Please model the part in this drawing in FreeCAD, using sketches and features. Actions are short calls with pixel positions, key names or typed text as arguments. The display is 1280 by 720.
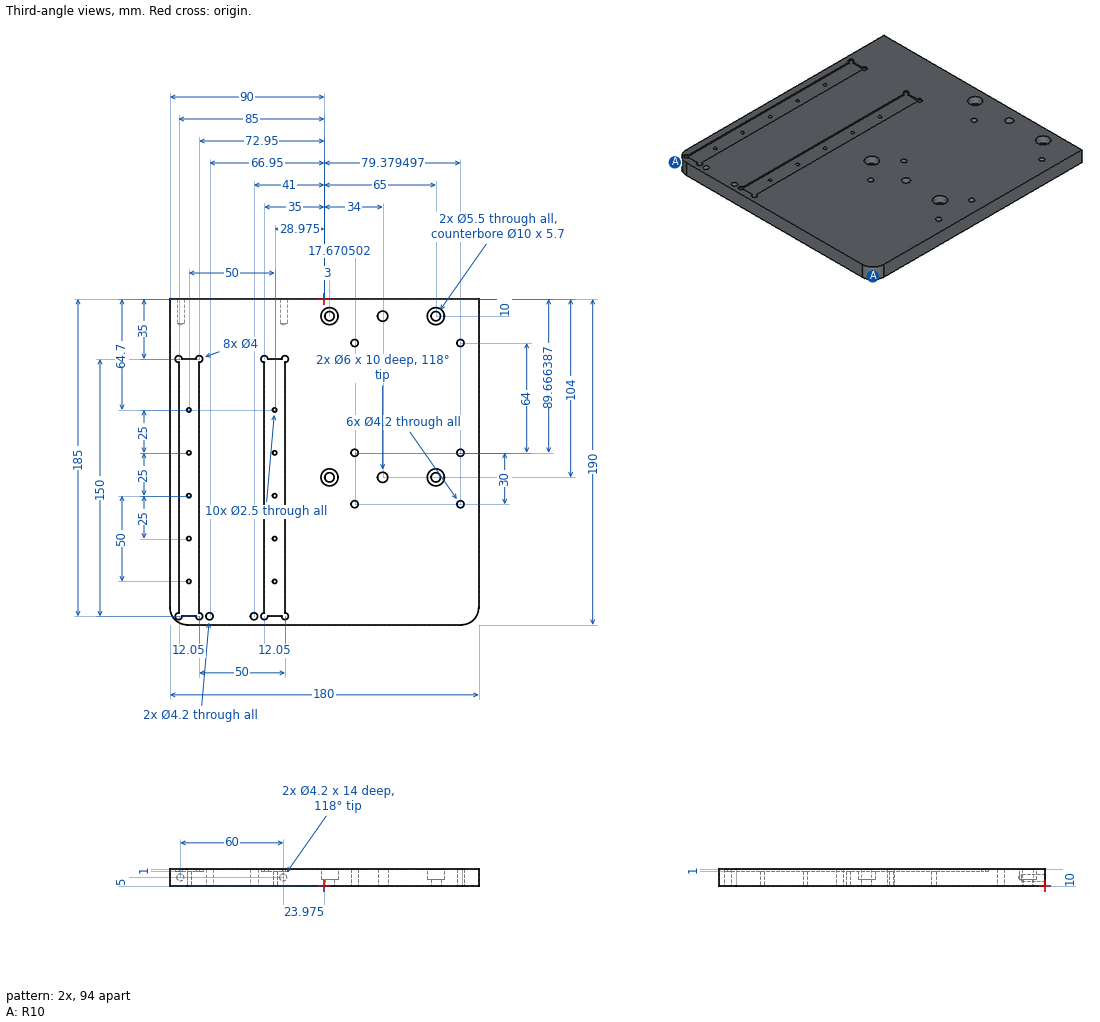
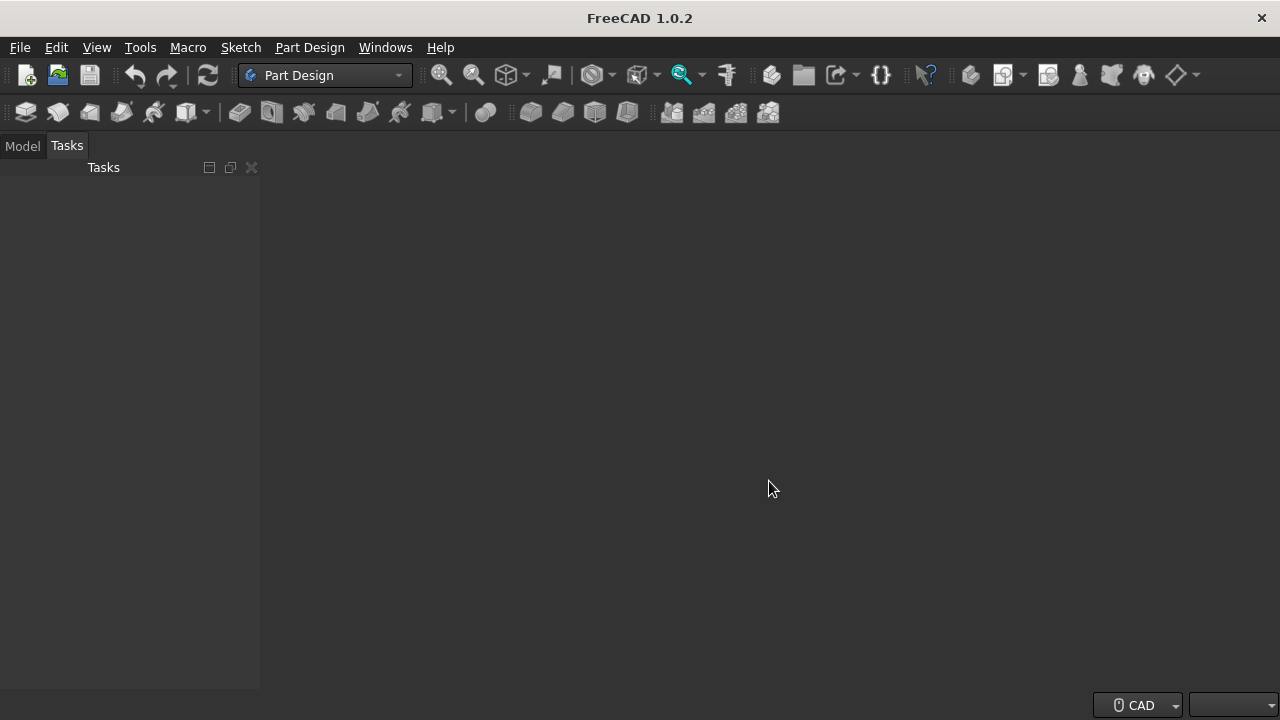
key(ctrl+n)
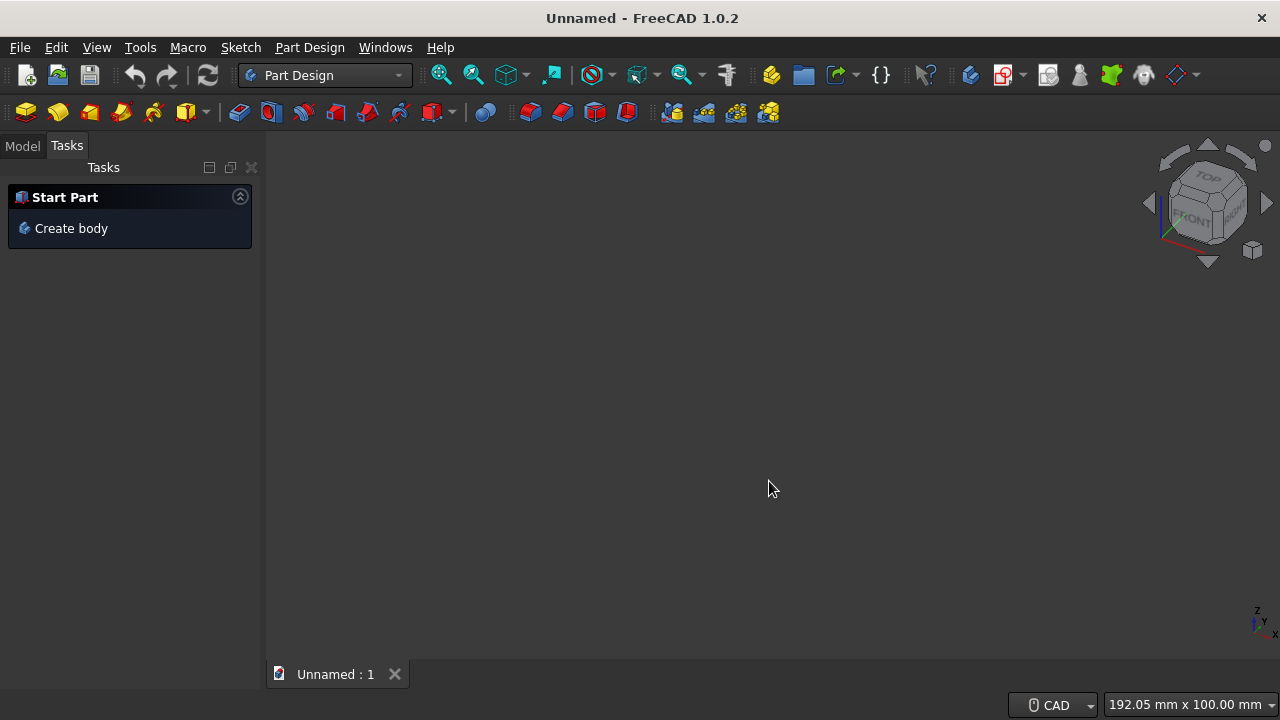
click(1004, 76)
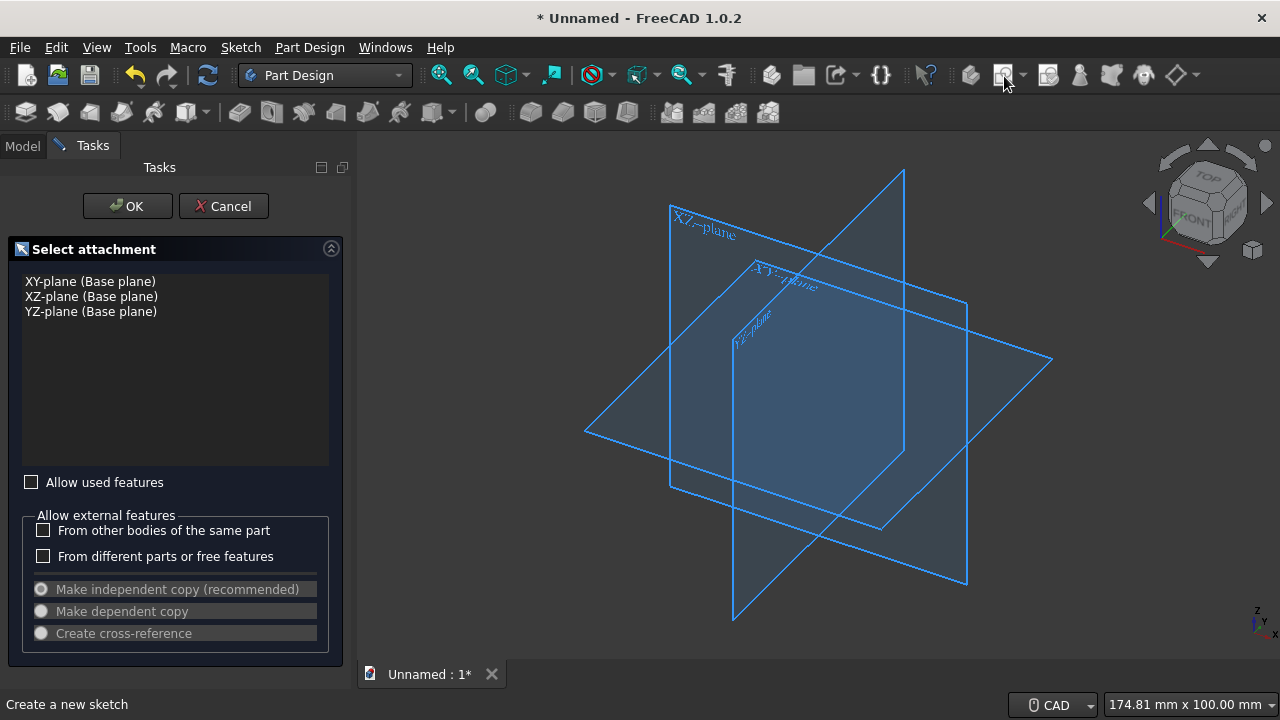
click(82, 282)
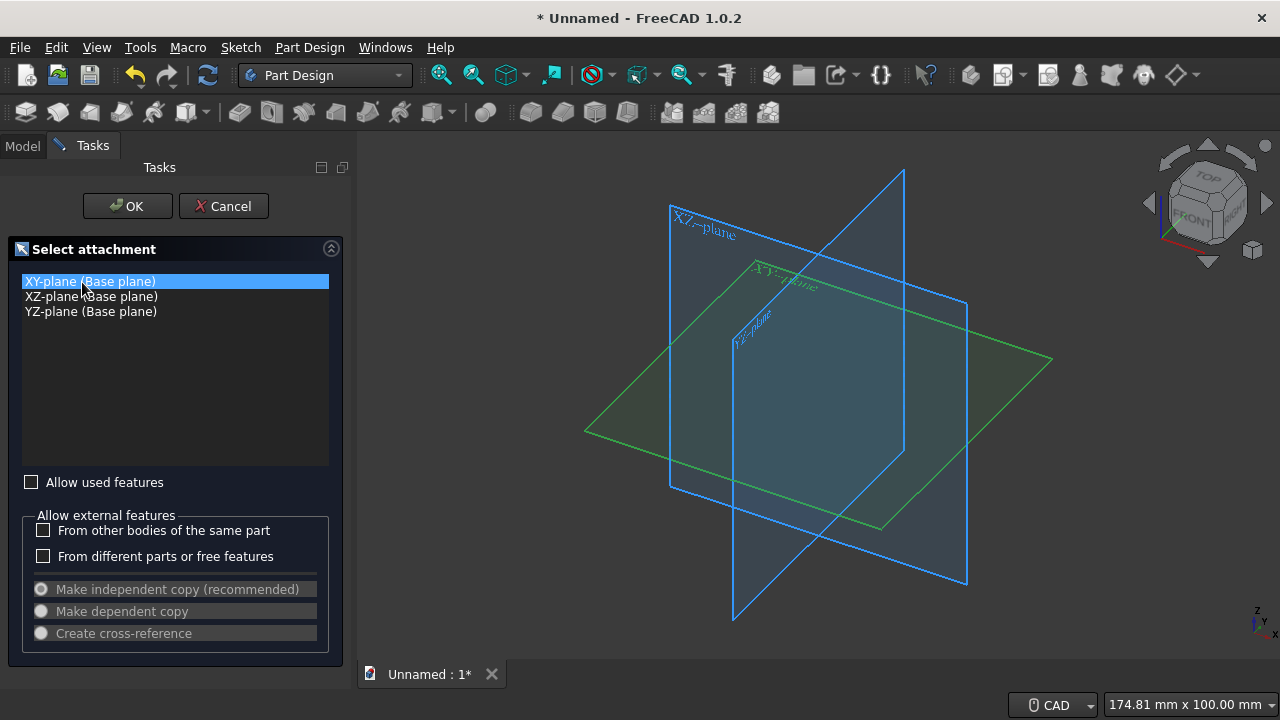
click(128, 206)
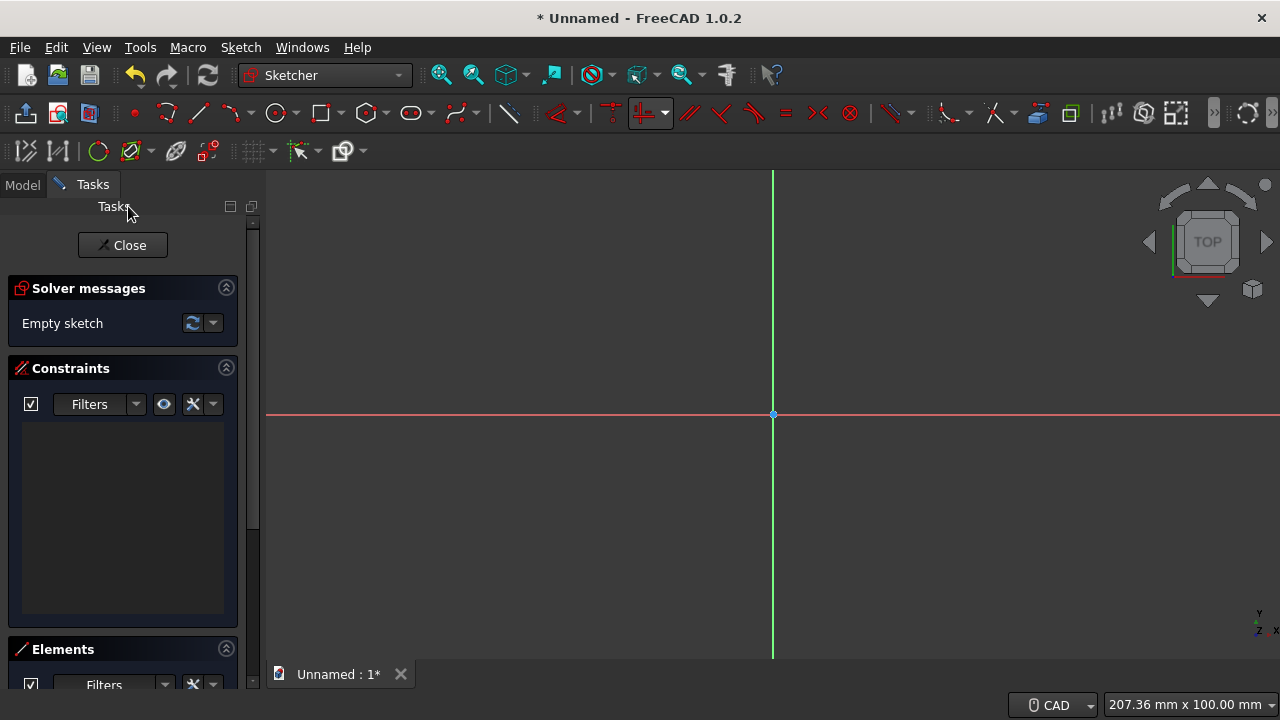
scroll(675, 214, down, 6)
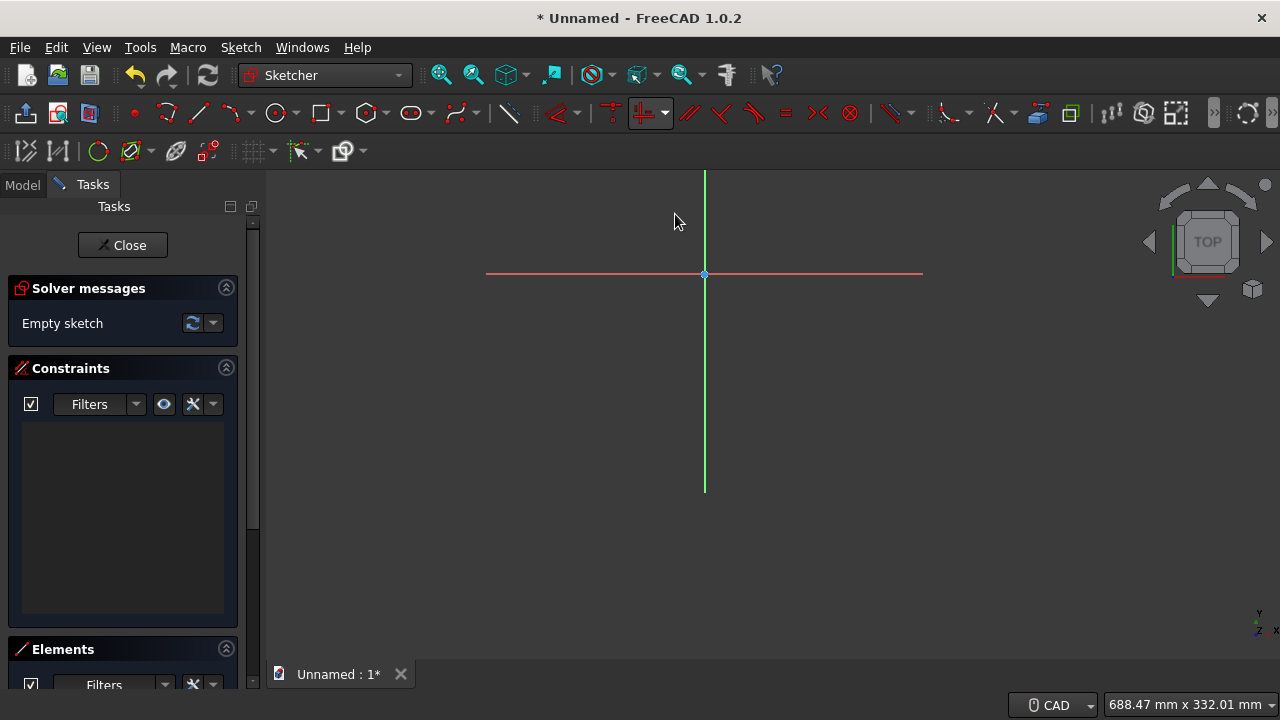
key(g)
key(r)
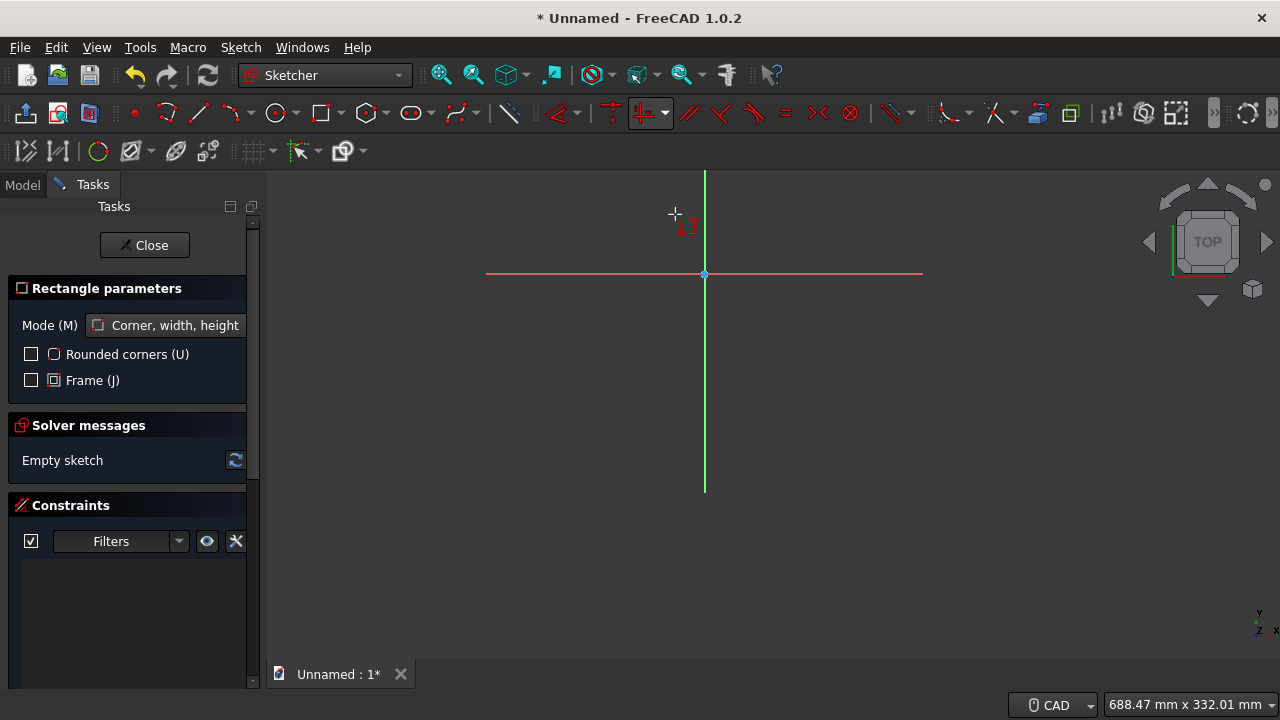
click(572, 274)
move(837, 554)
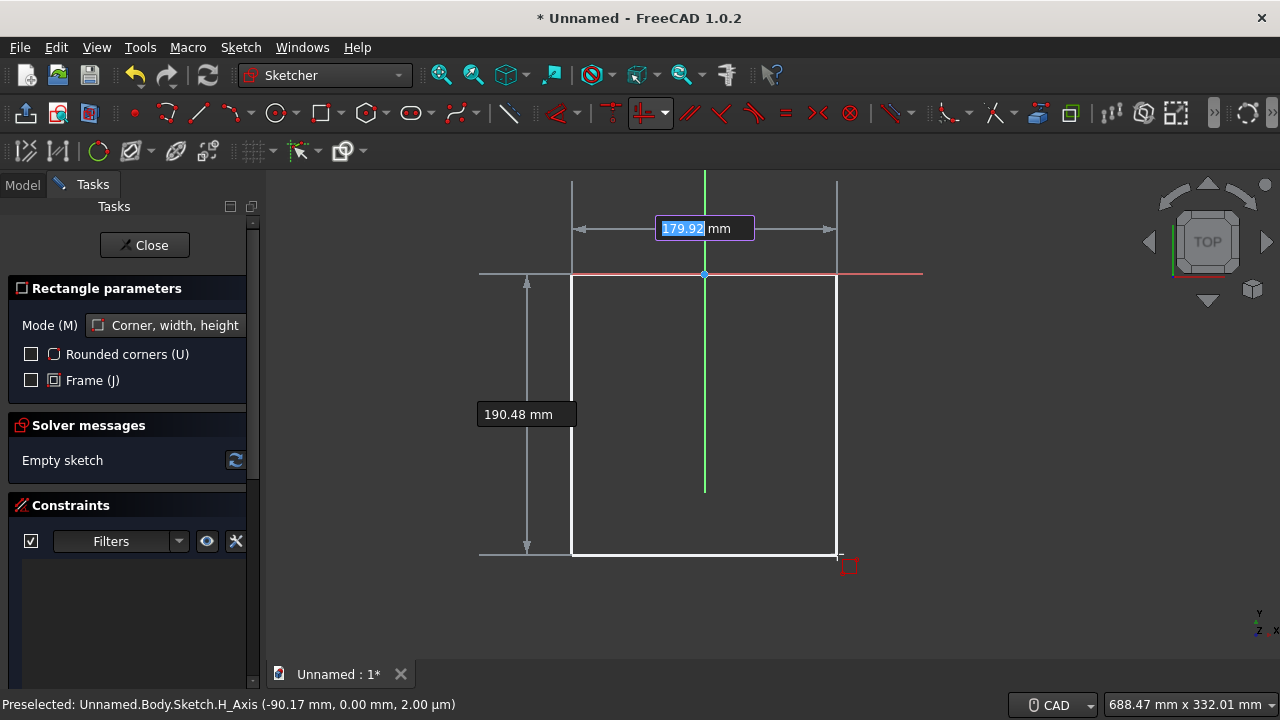
text(180)
key(Tab)
text(190)
key(Return)
key(Escape)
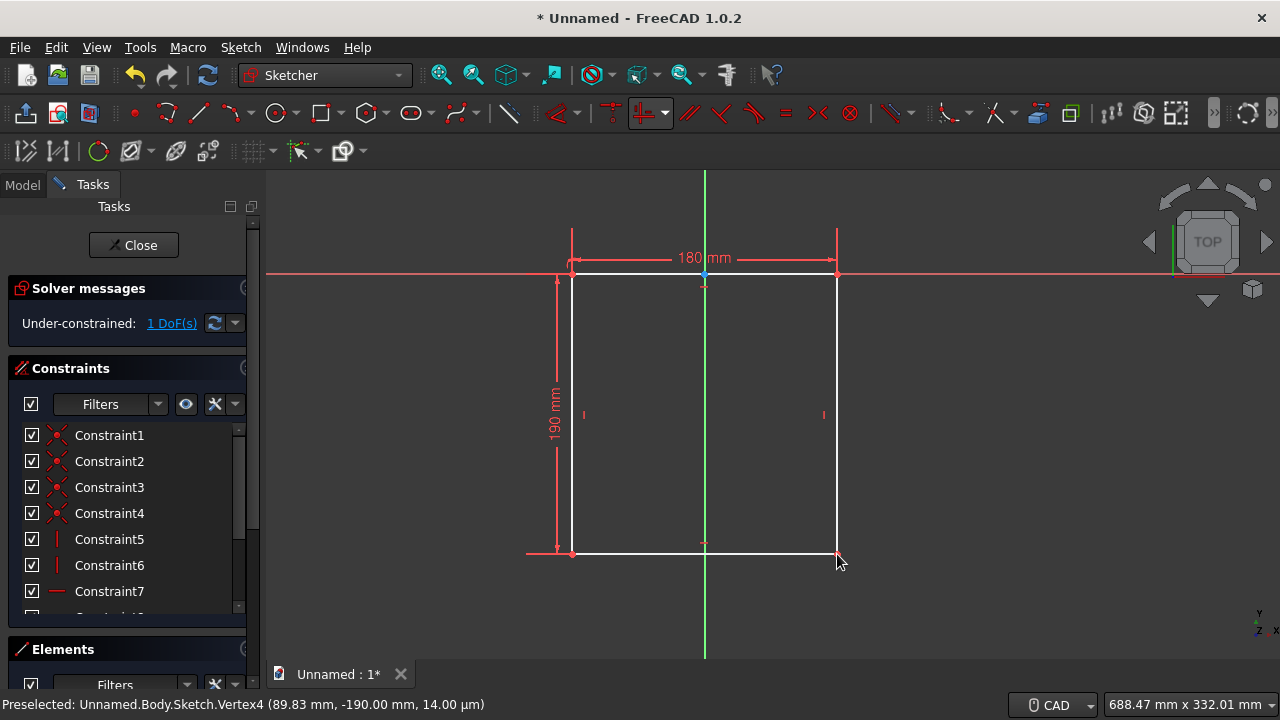
click(572, 274)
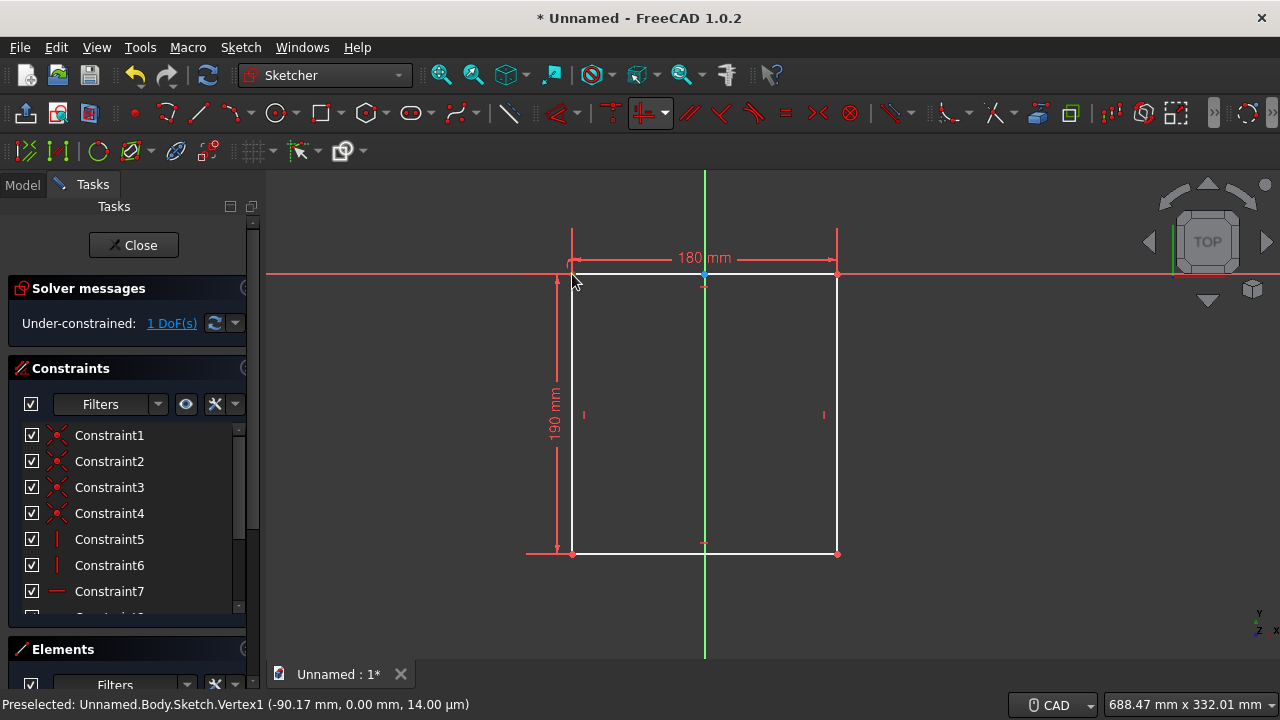
key(l)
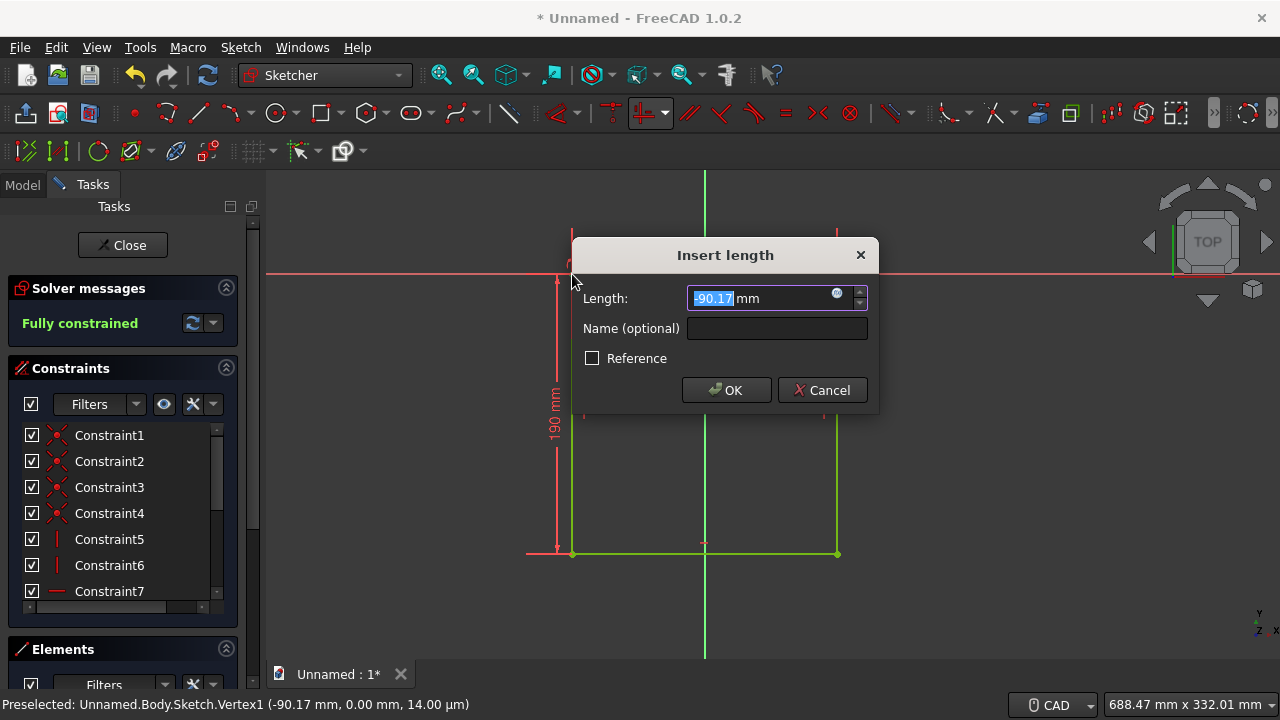
text(-90)
key(Return)